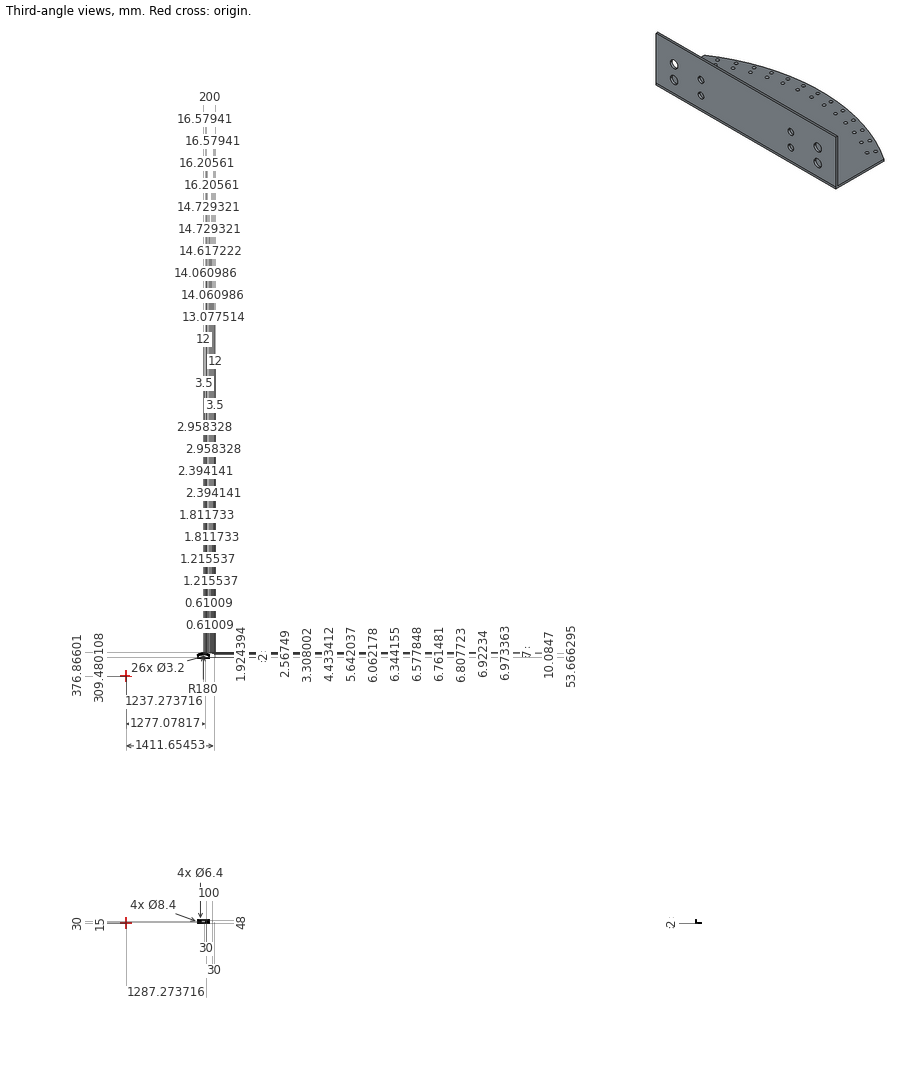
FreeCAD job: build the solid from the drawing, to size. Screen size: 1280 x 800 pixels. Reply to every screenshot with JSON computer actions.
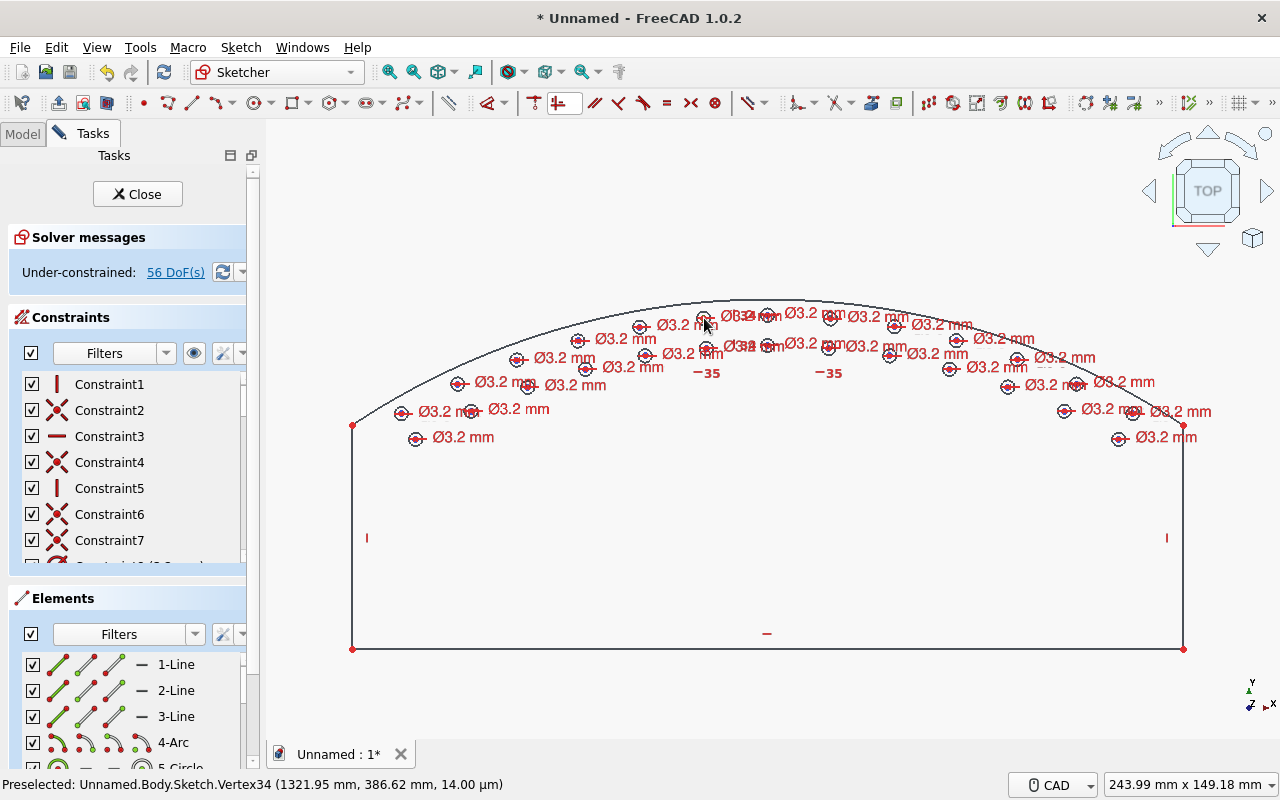
{"action": "left_click", "coordinate": [576, 104]}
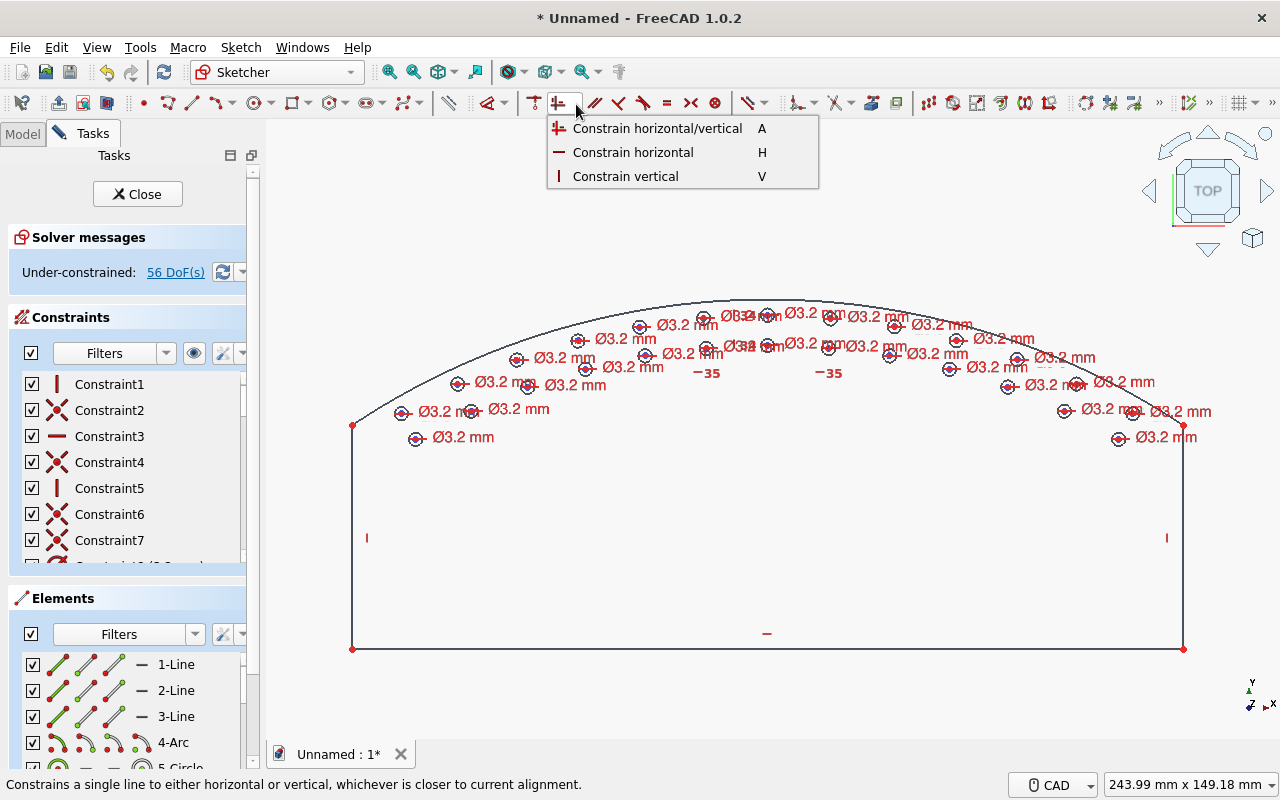
{"action": "left_click", "coordinate": [683, 152]}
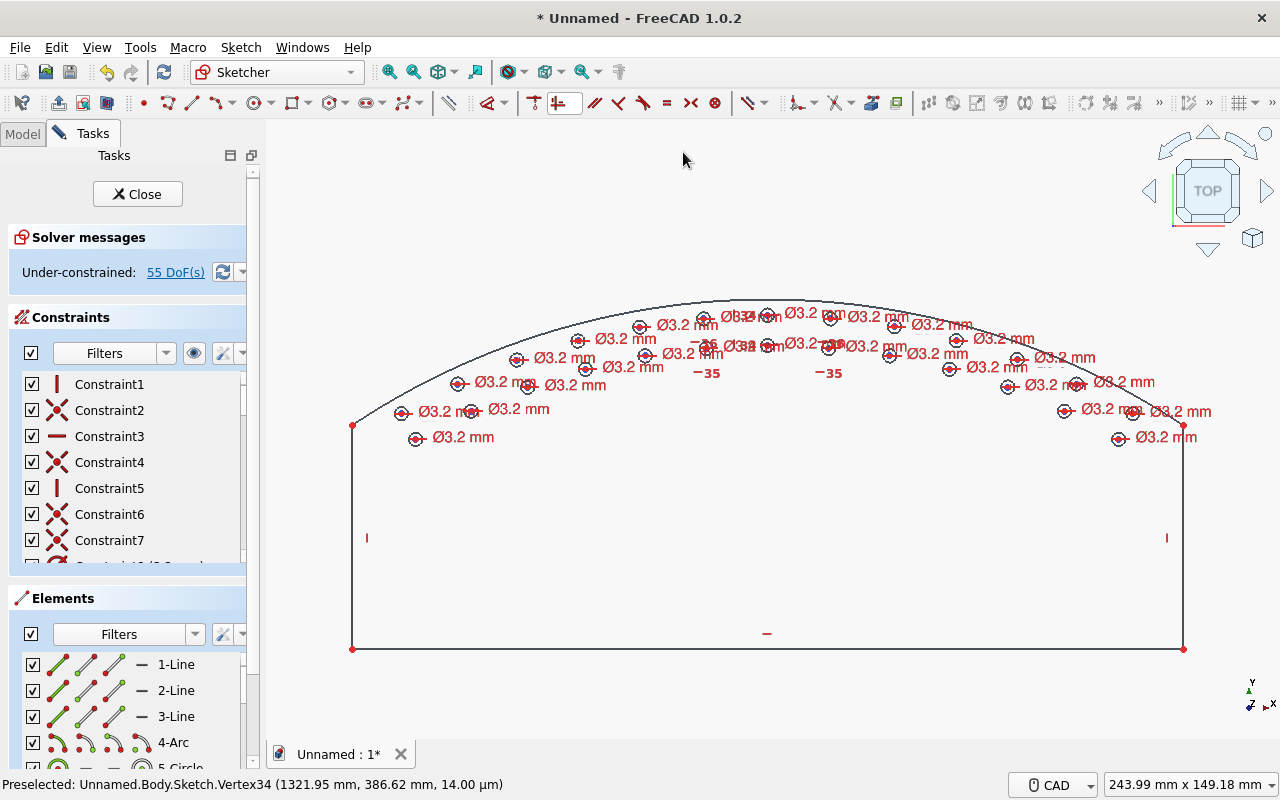
{"action": "left_click", "coordinate": [488, 104]}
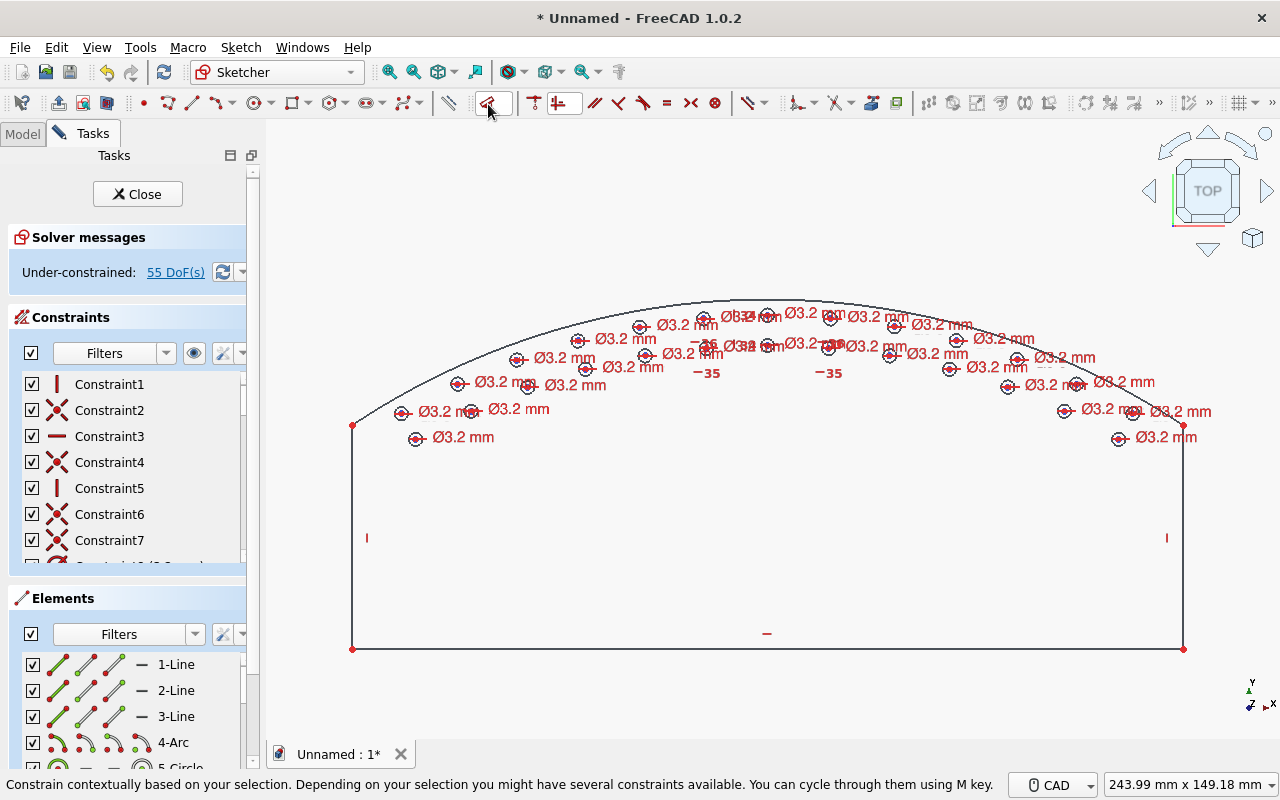
{"action": "left_click", "coordinate": [942, 320]}
{"action": "left_click", "coordinate": [949, 289]}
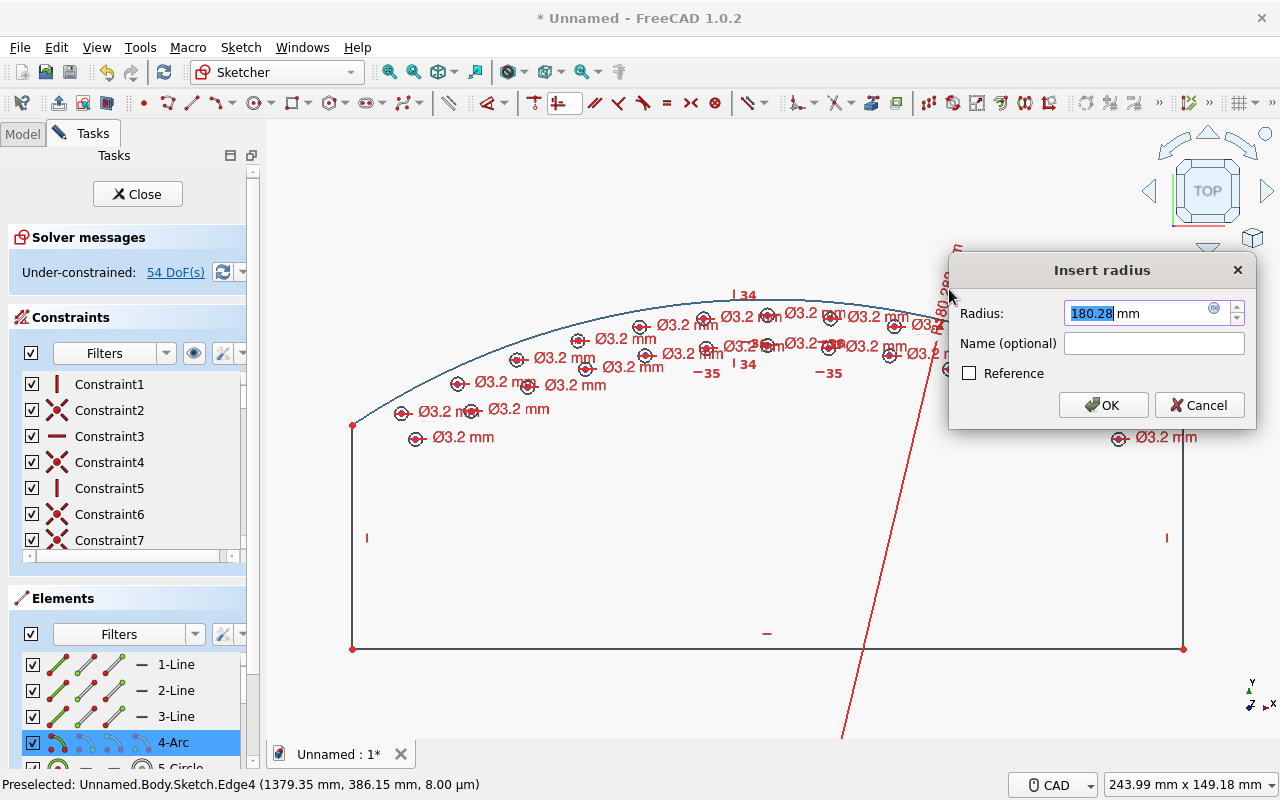
{"action": "type", "text": "180"}
{"action": "key", "text": "Return"}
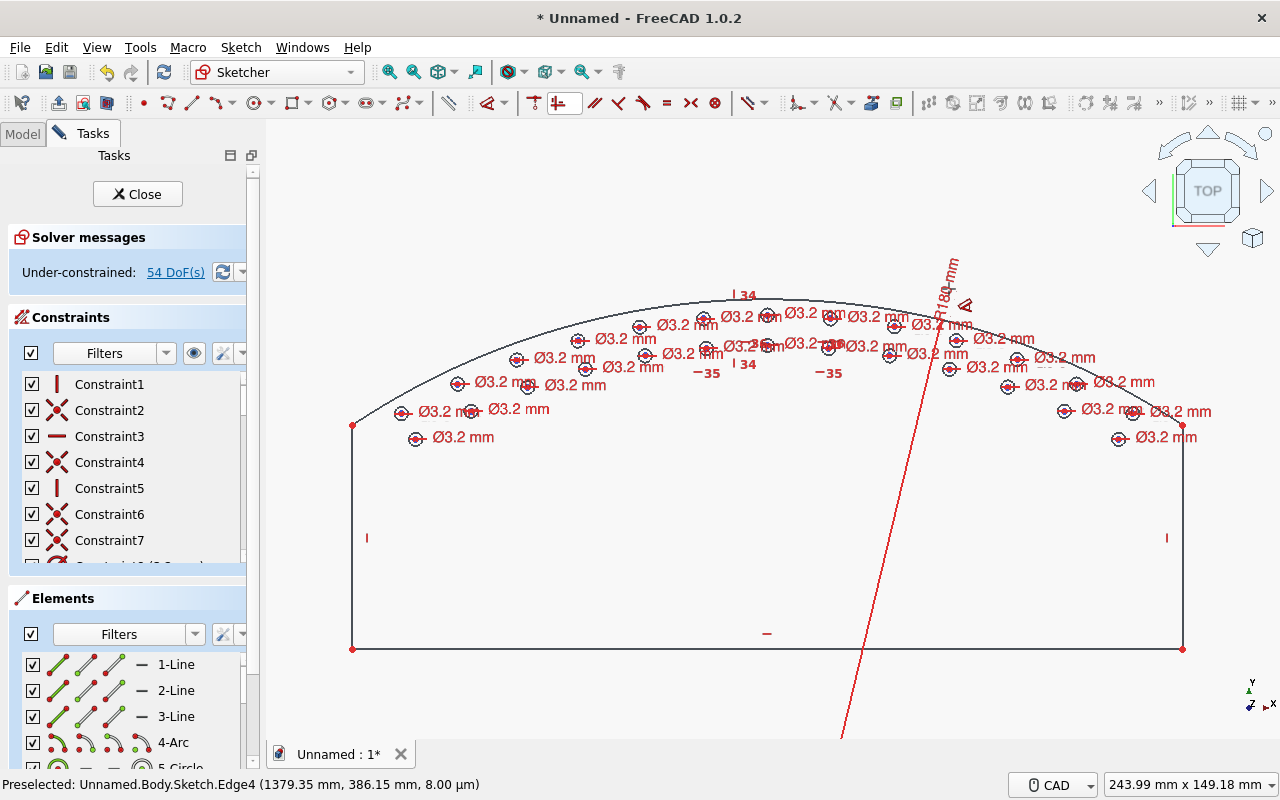
{"action": "scroll", "coordinate": [768, 345], "scroll_direction": "up", "scroll_amount": 2}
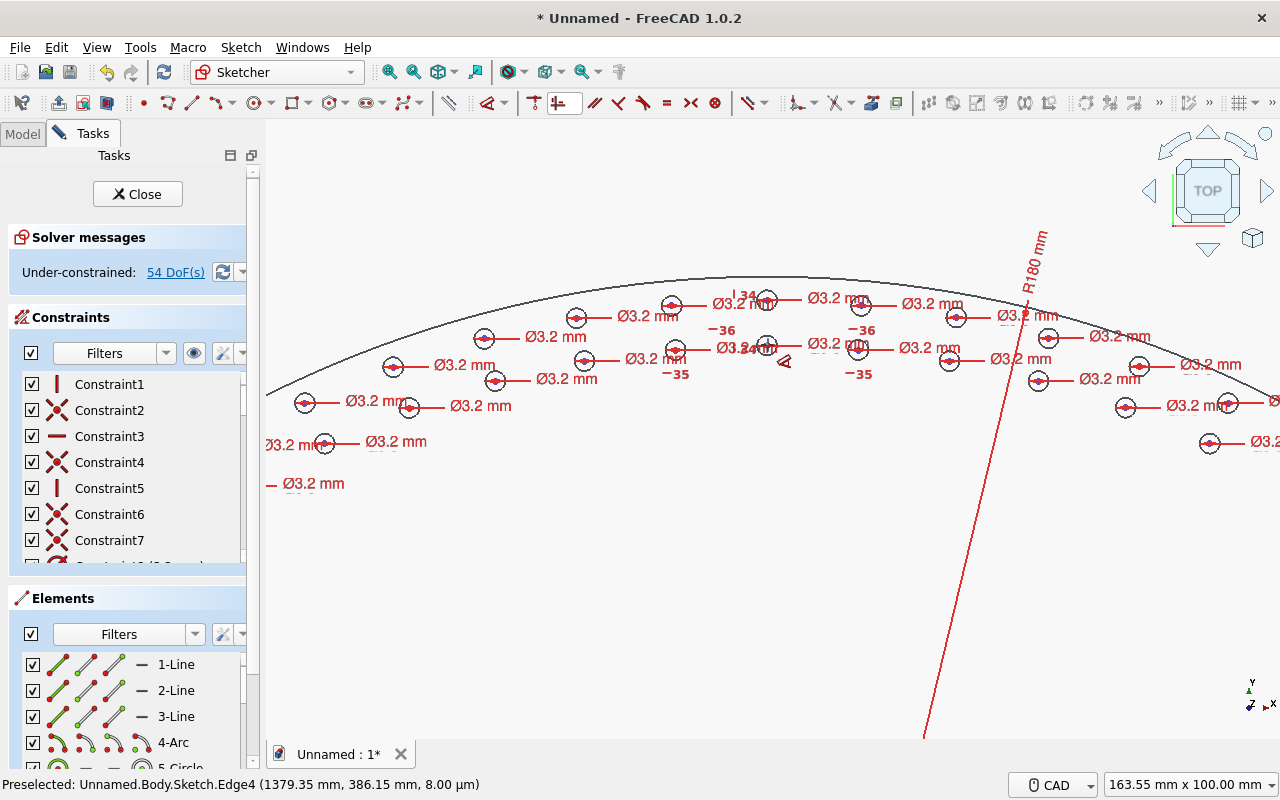
{"action": "left_click", "coordinate": [767, 346]}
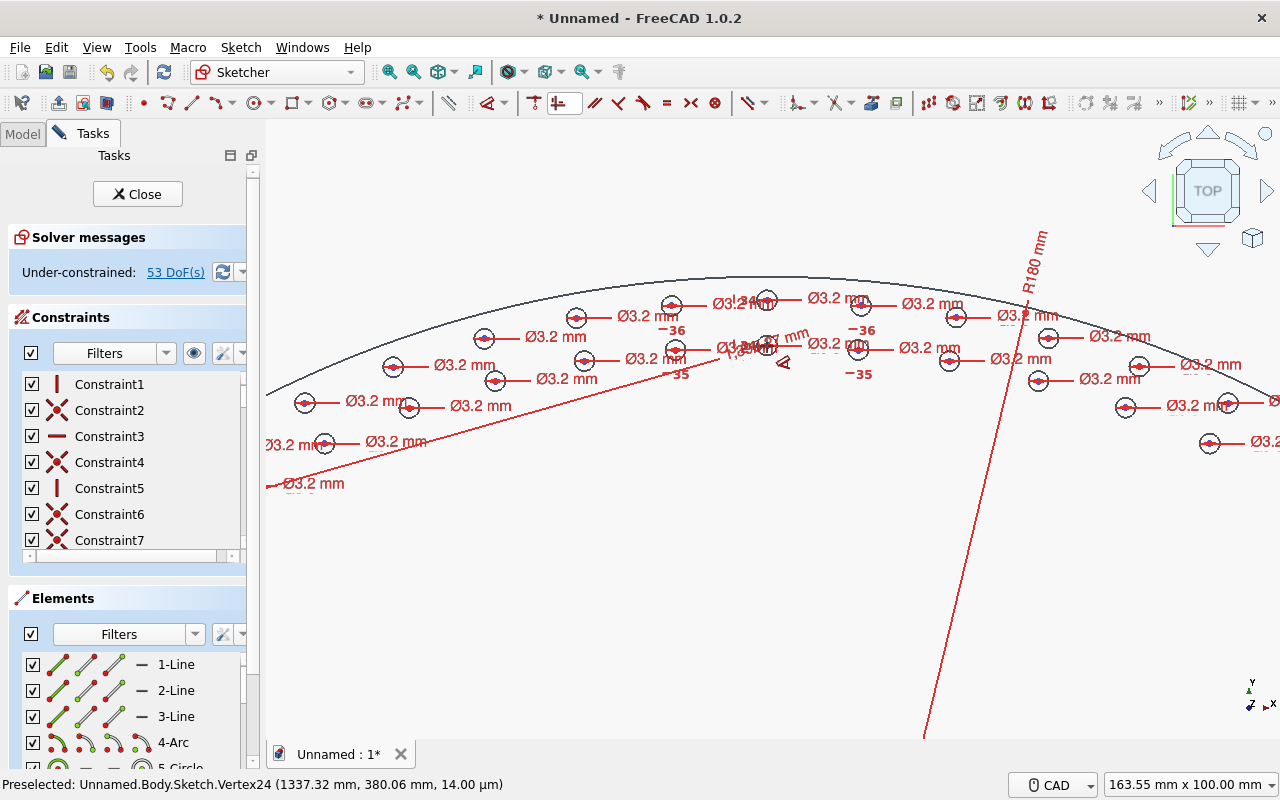
{"action": "left_click", "coordinate": [767, 300]}
{"action": "left_click", "coordinate": [801, 323]}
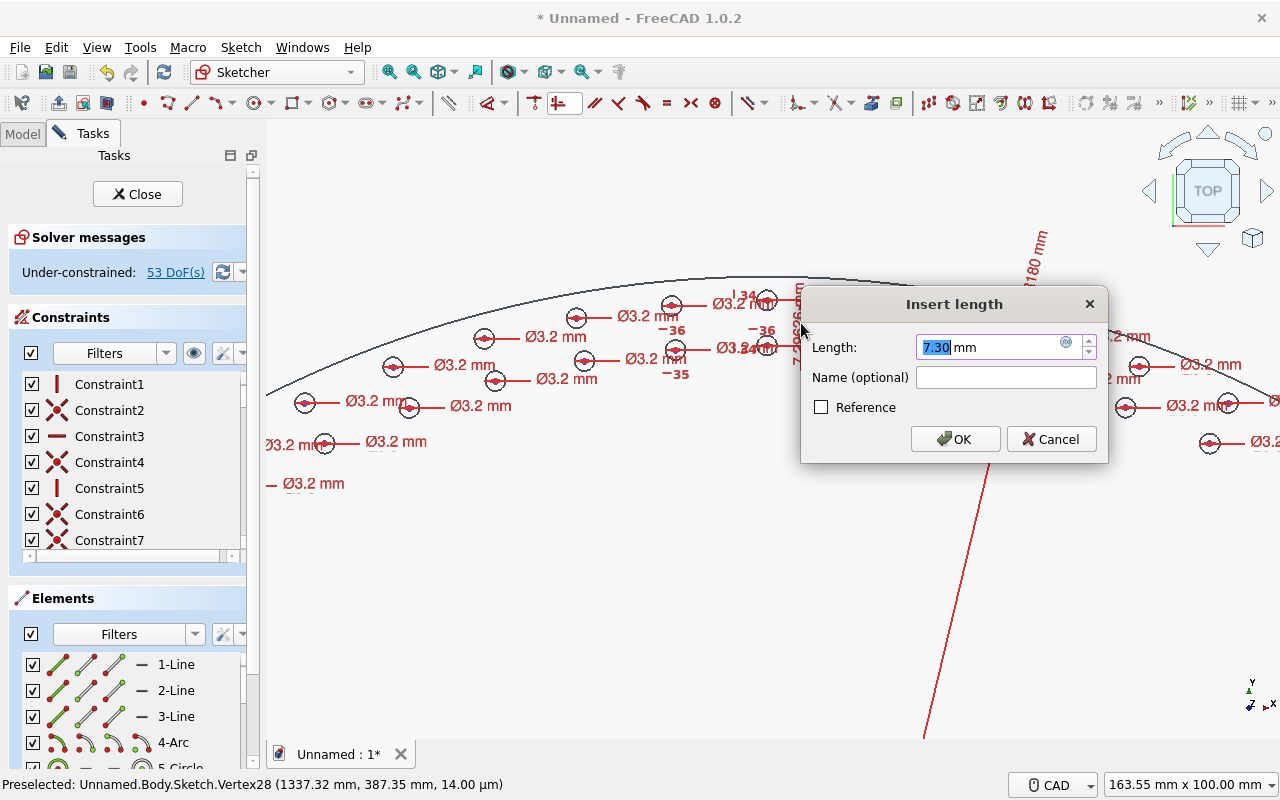
{"action": "type", "text": "7"}
{"action": "key", "text": "Return"}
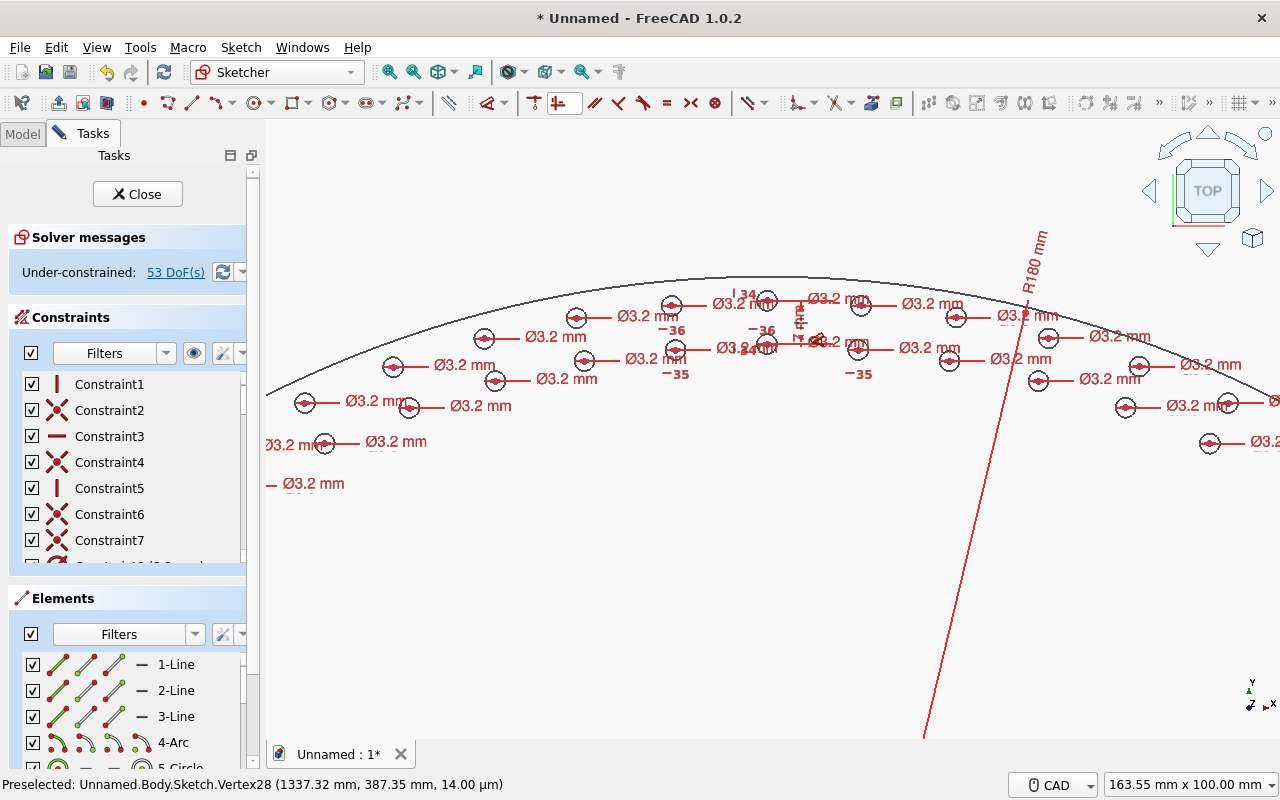
{"action": "scroll", "coordinate": [654, 342], "scroll_direction": "down", "scroll_amount": 4}